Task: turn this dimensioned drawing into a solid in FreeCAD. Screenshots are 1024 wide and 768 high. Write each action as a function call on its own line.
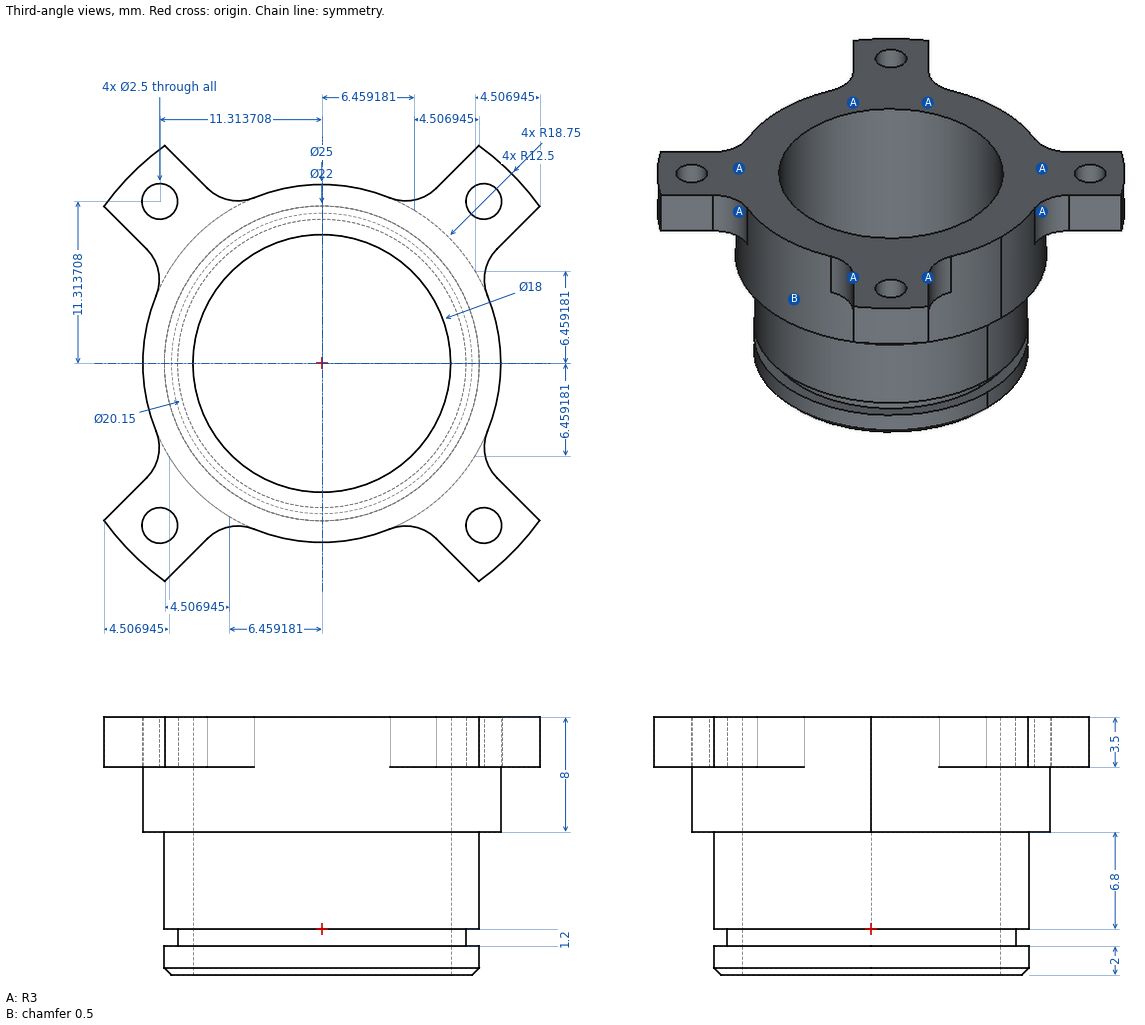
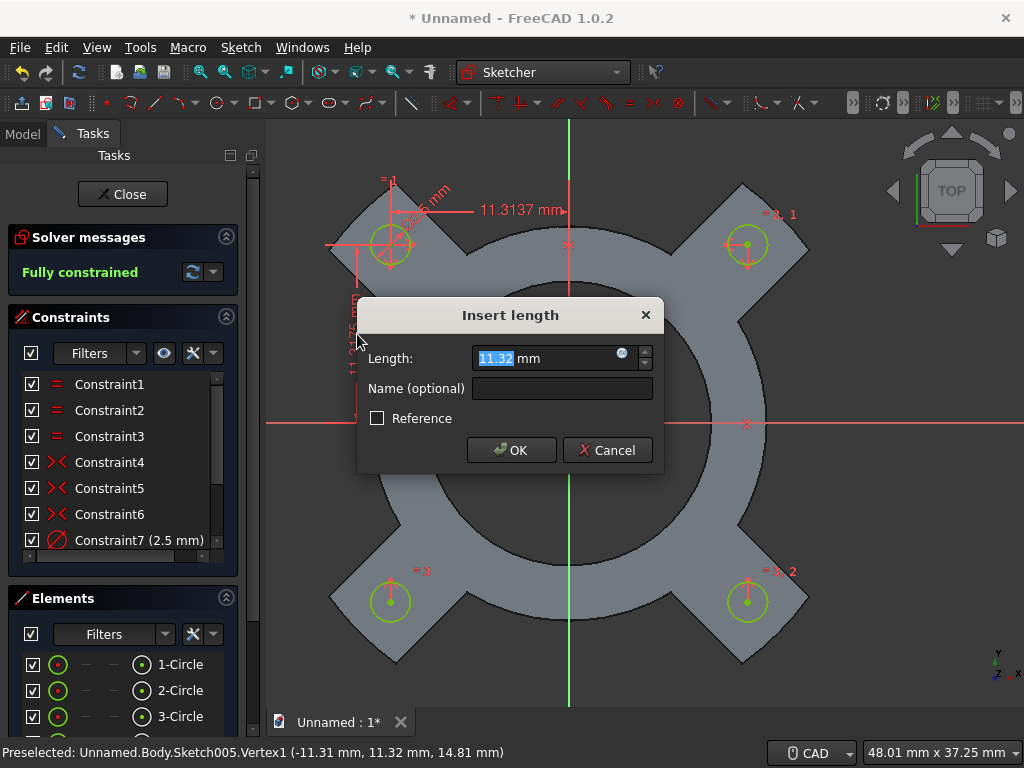
text(11.313708)
key(Return)
key(Escape)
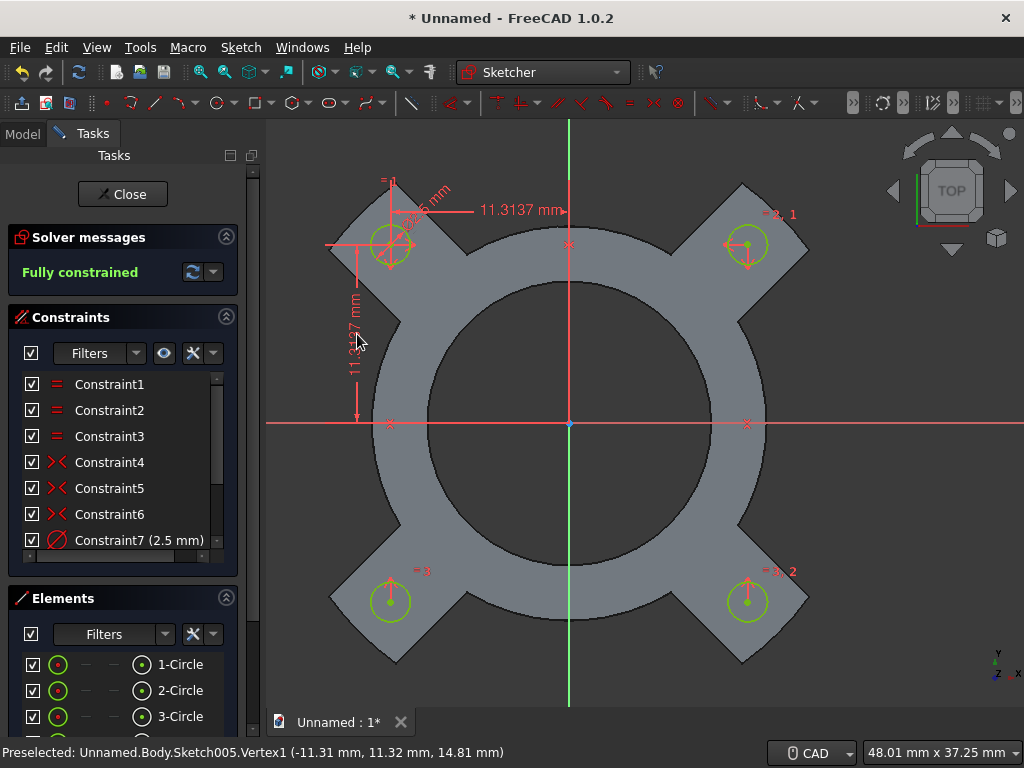
click(123, 194)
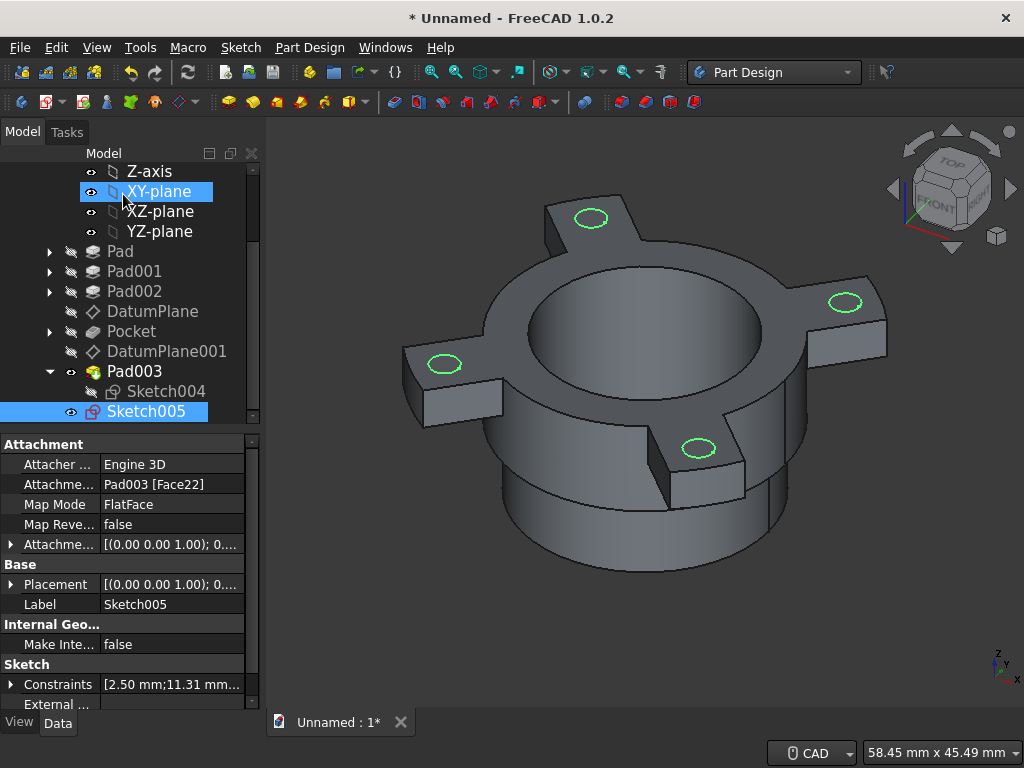
click(420, 102)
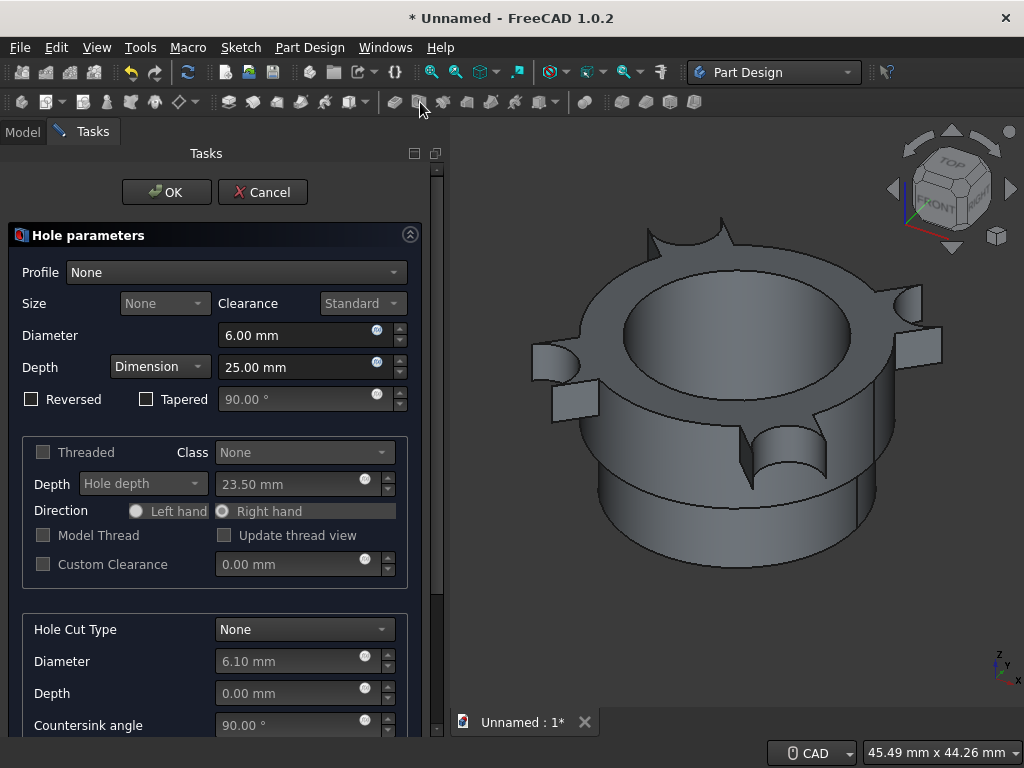
triple_click(305, 335)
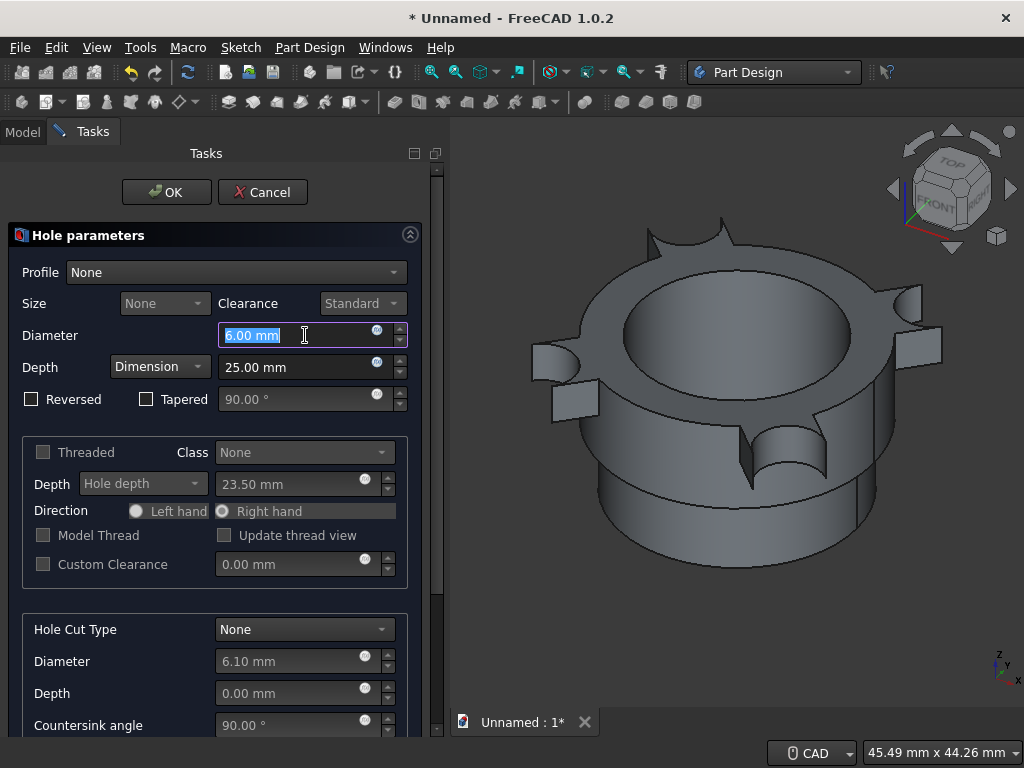
text(2.5)
key(Tab)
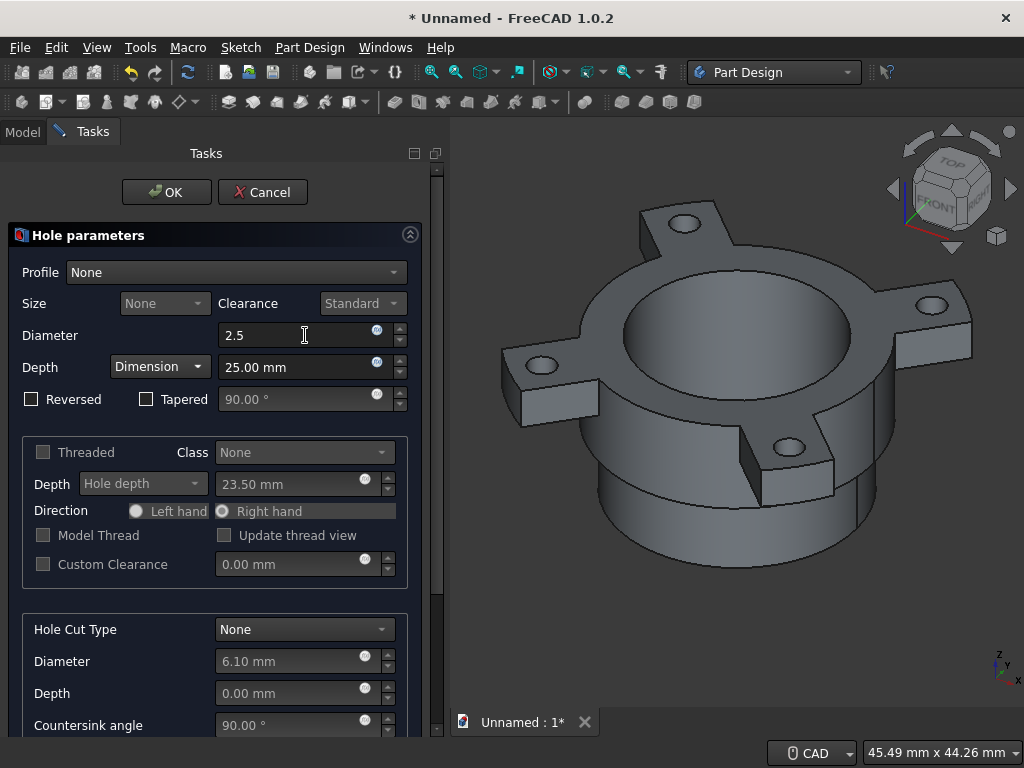
click(161, 366)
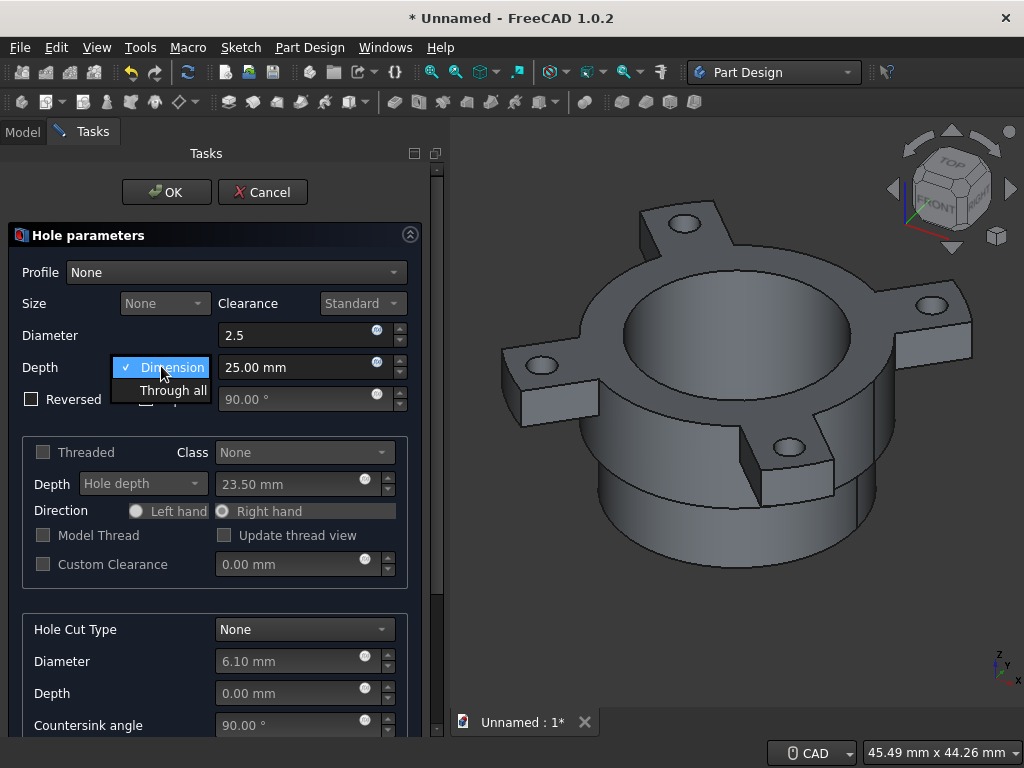
click(160, 390)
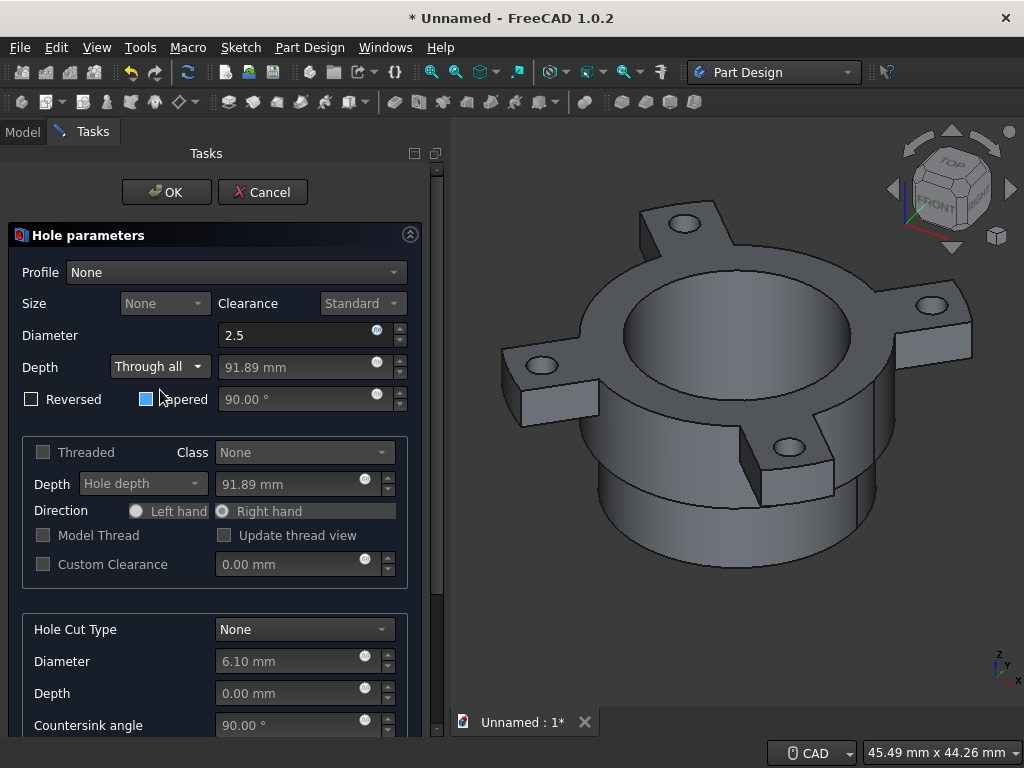
click(167, 192)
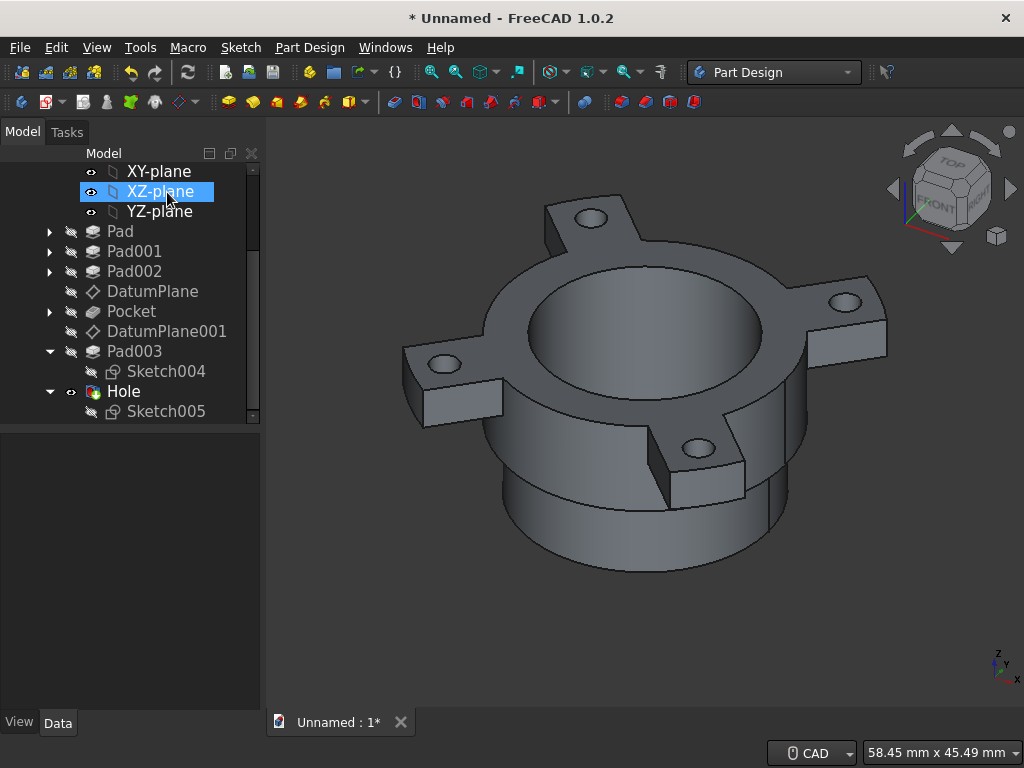
key(0)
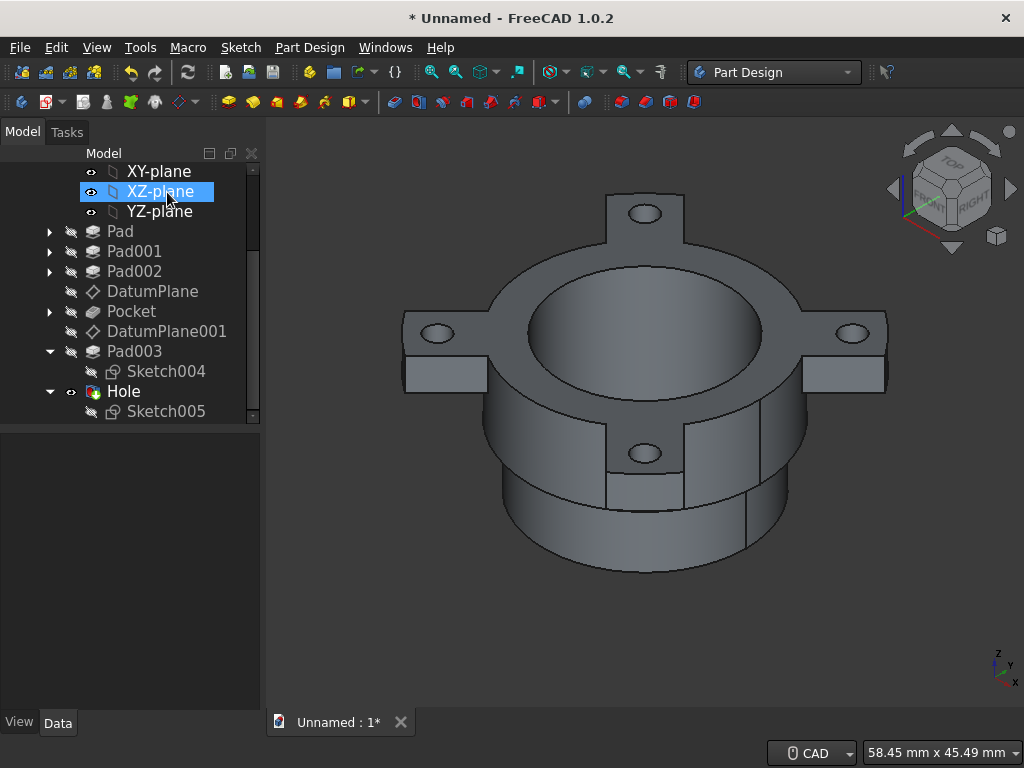
key(2)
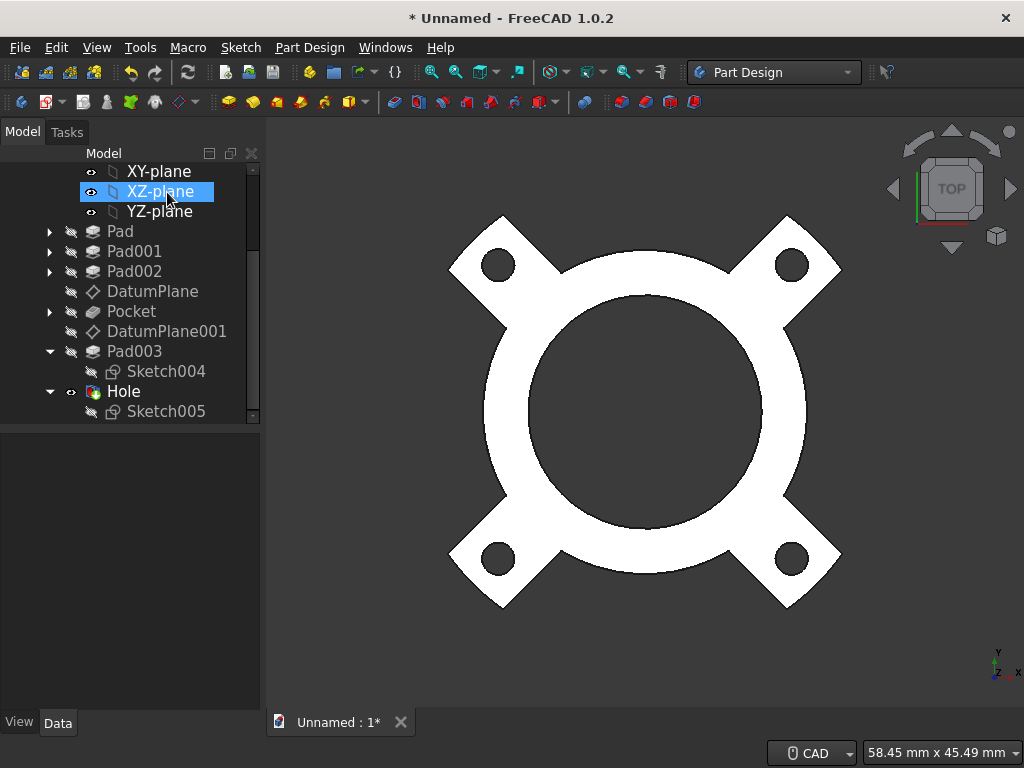
key(1)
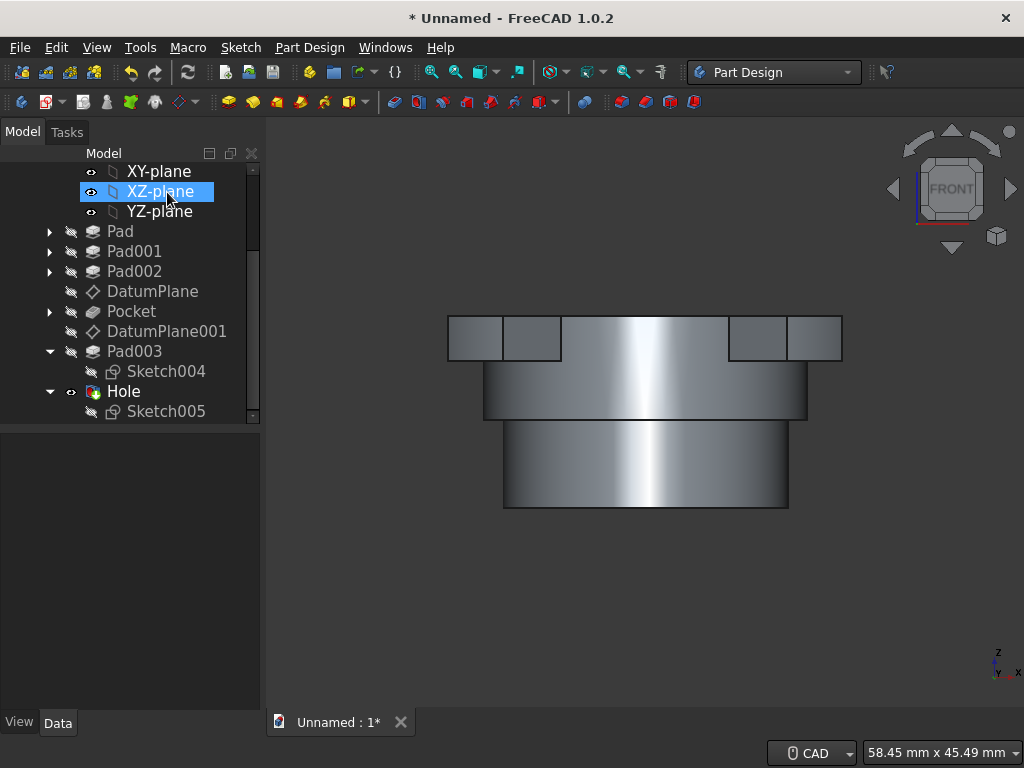
key(3)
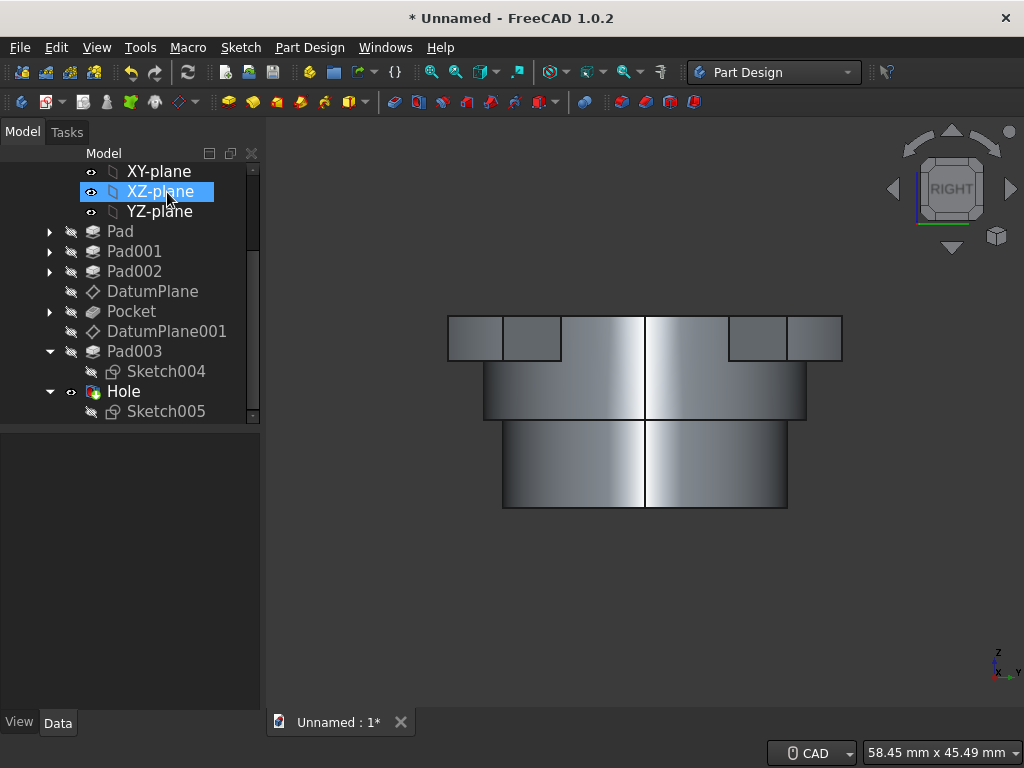
key(5)